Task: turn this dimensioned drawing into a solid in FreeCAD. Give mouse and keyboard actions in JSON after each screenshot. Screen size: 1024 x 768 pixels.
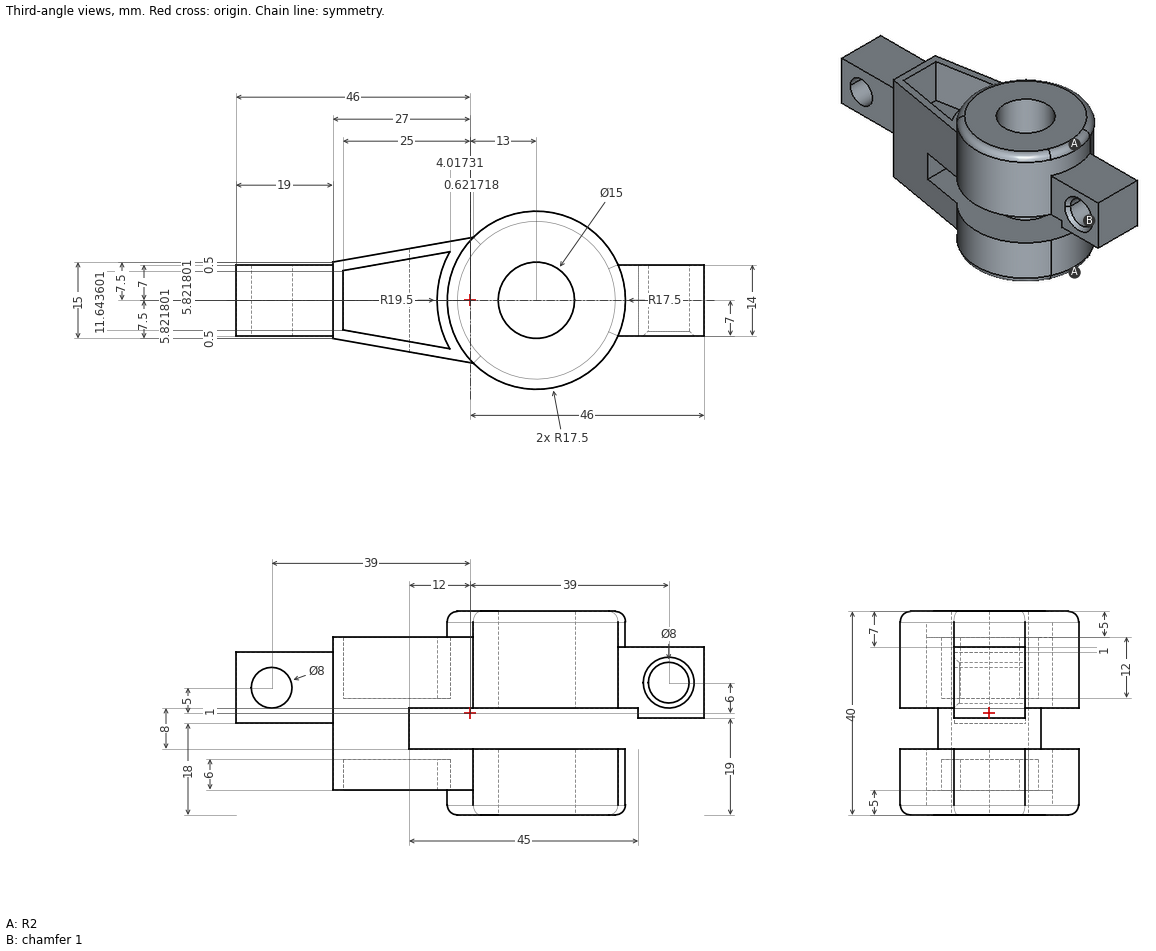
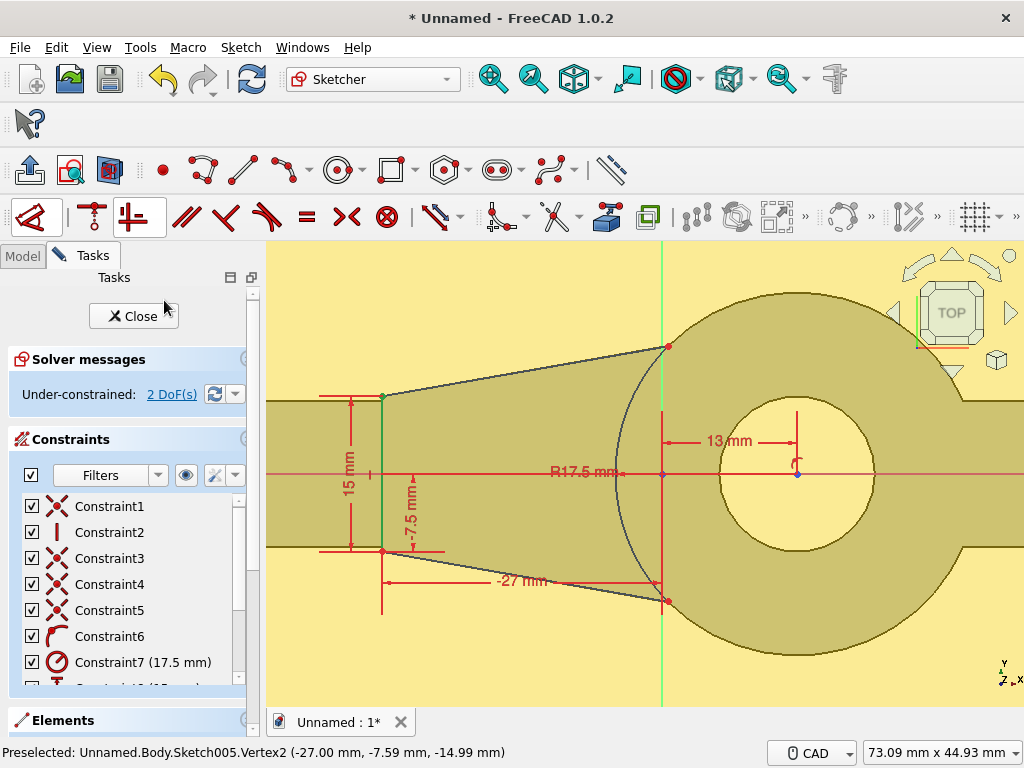
{"action": "scroll", "coordinate": [668, 602], "scroll_direction": "up", "scroll_amount": 10}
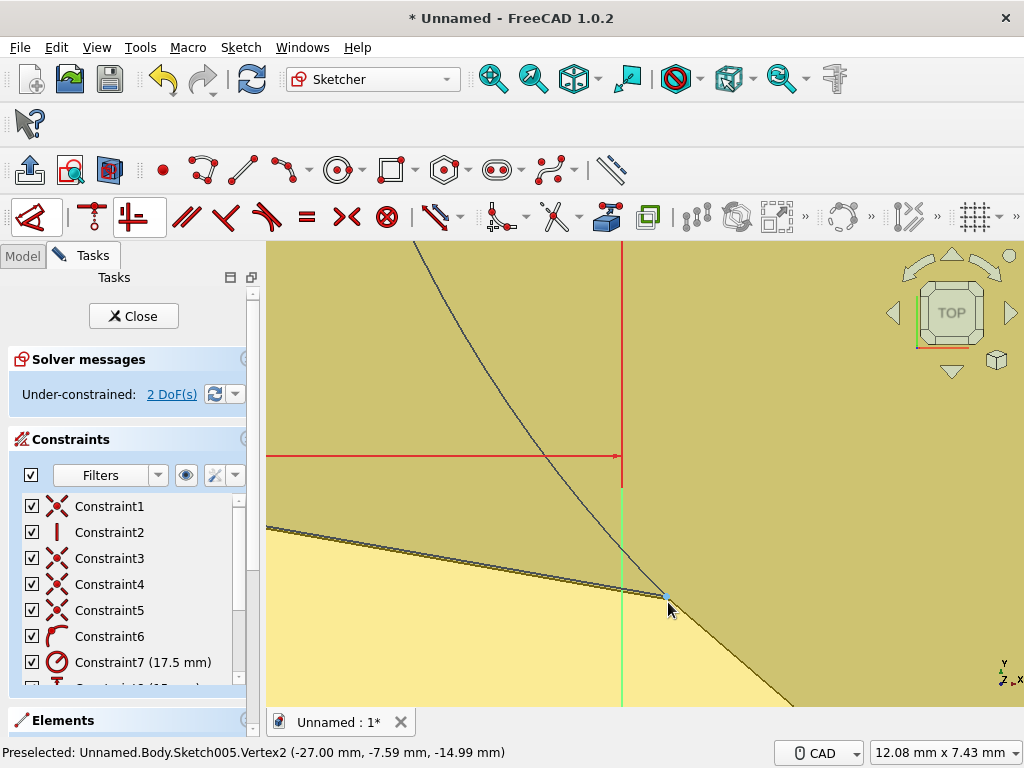
{"action": "left_click", "coordinate": [666, 596]}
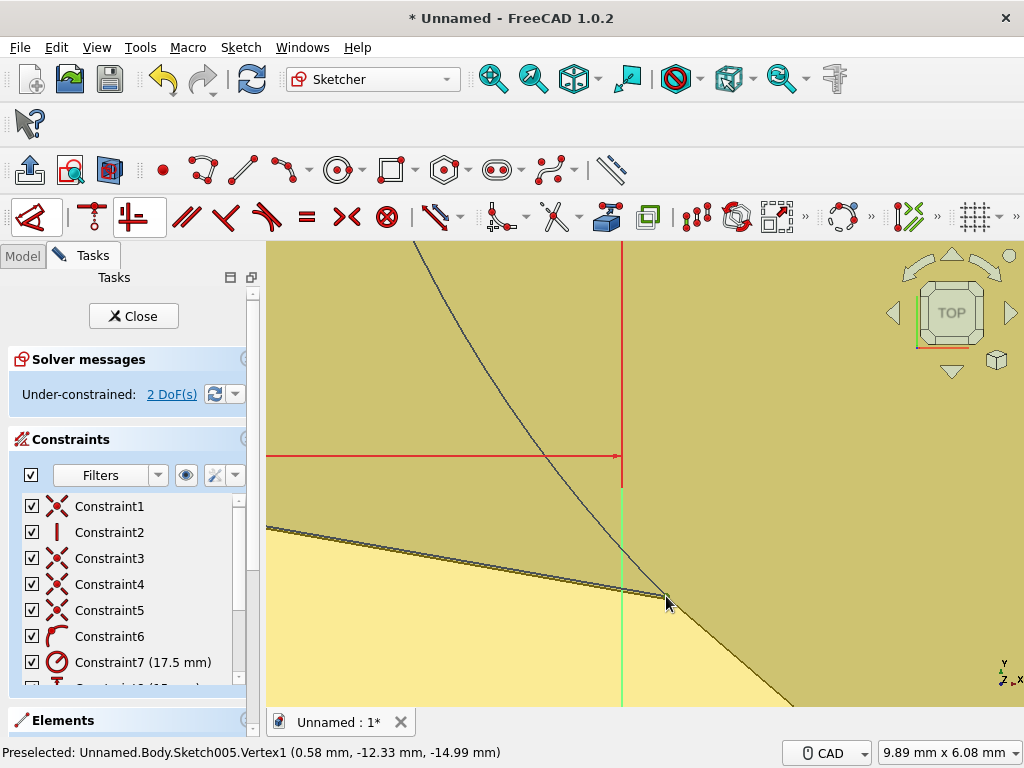
{"action": "key", "text": "l"}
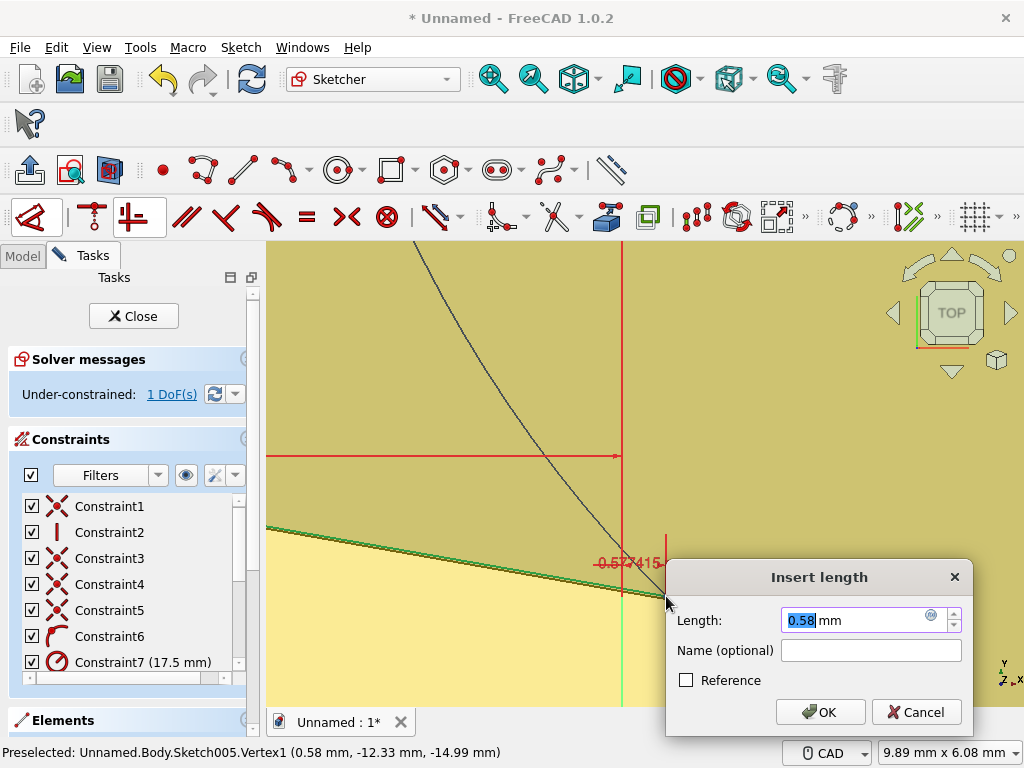
{"action": "type", "text": "0.621718"}
{"action": "key", "text": "Return"}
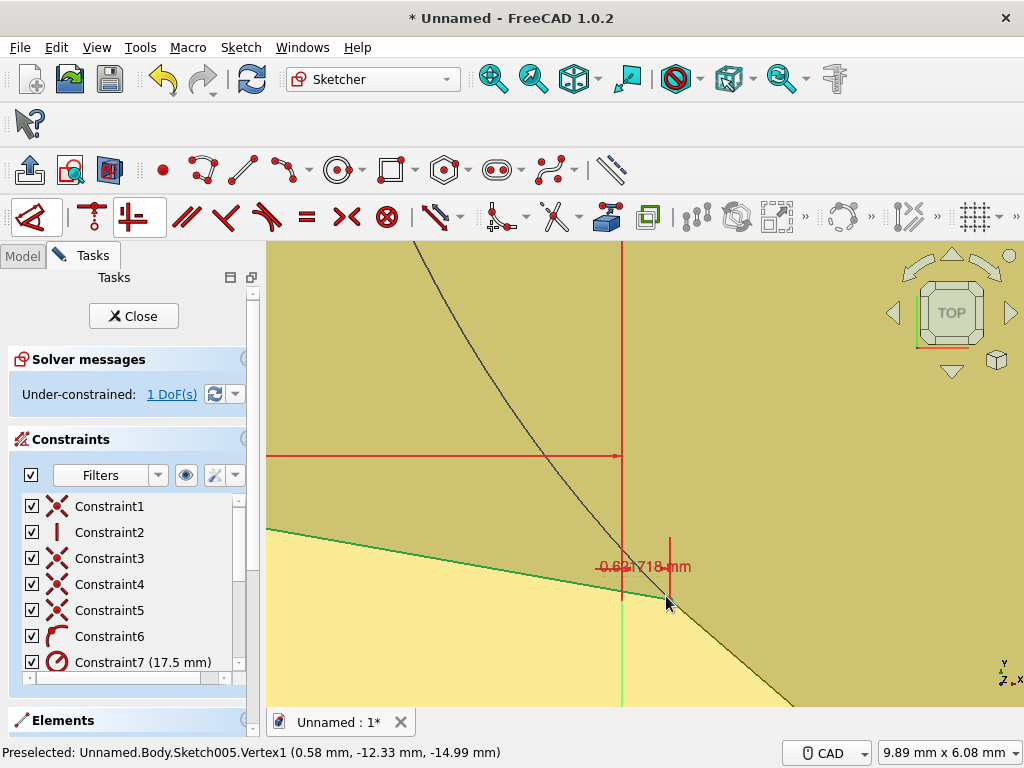
{"action": "scroll", "coordinate": [768, 637], "scroll_direction": "down", "scroll_amount": 9}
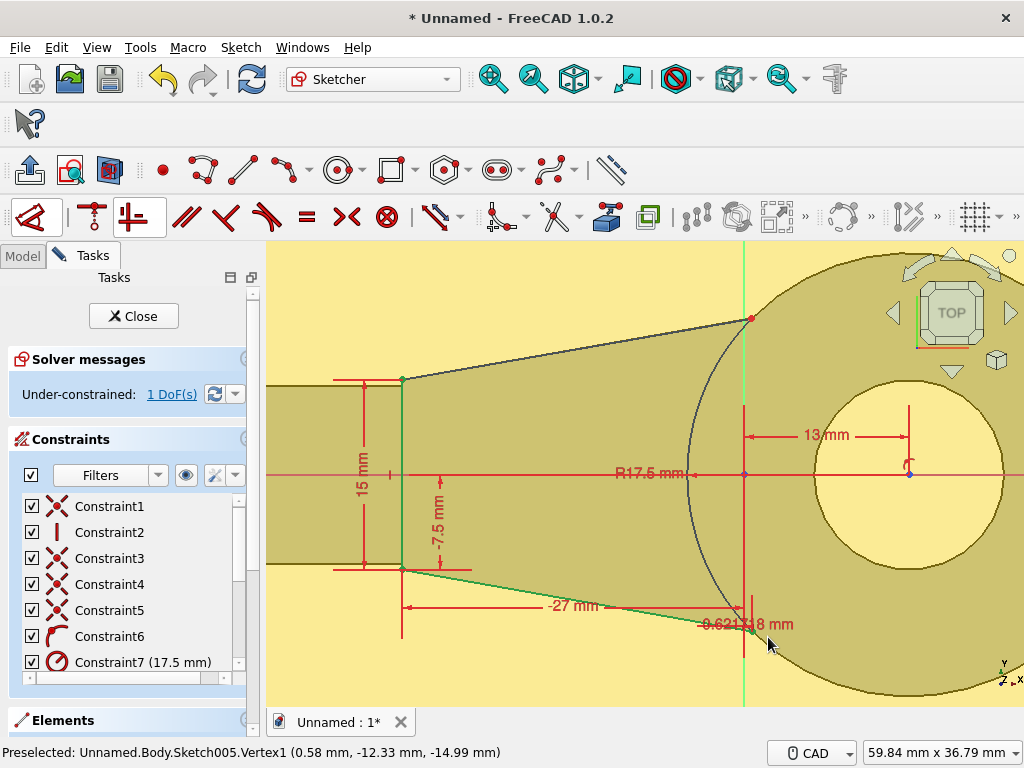
{"action": "scroll", "coordinate": [752, 319], "scroll_direction": "up", "scroll_amount": 9}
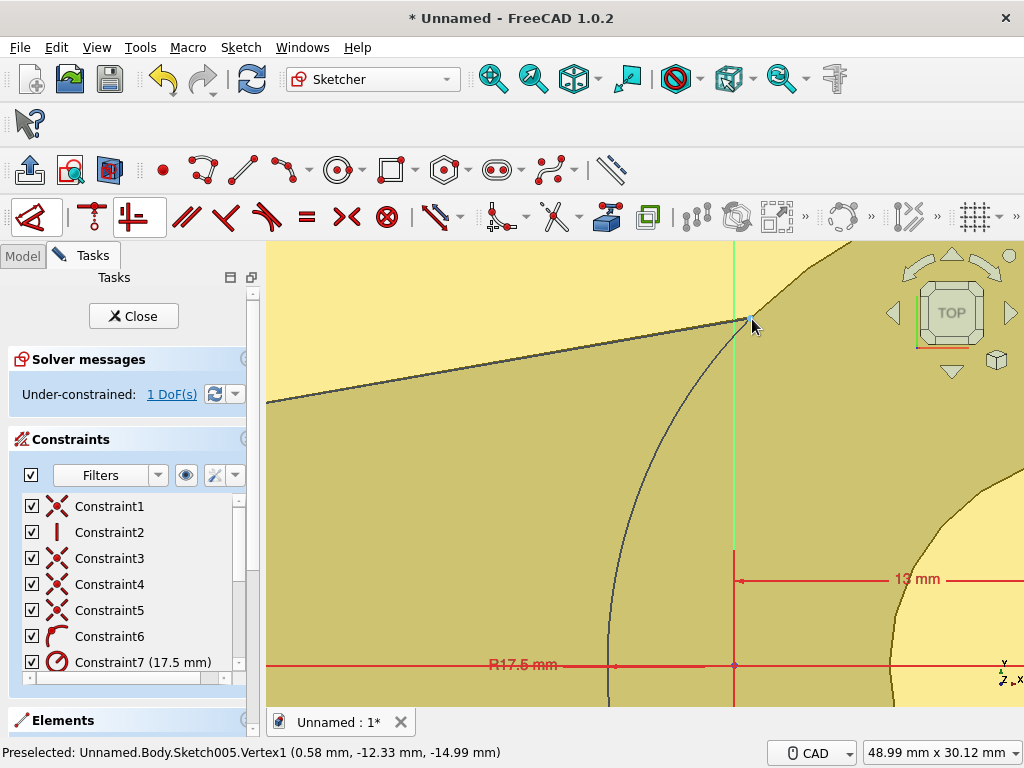
{"action": "left_click", "coordinate": [747, 317]}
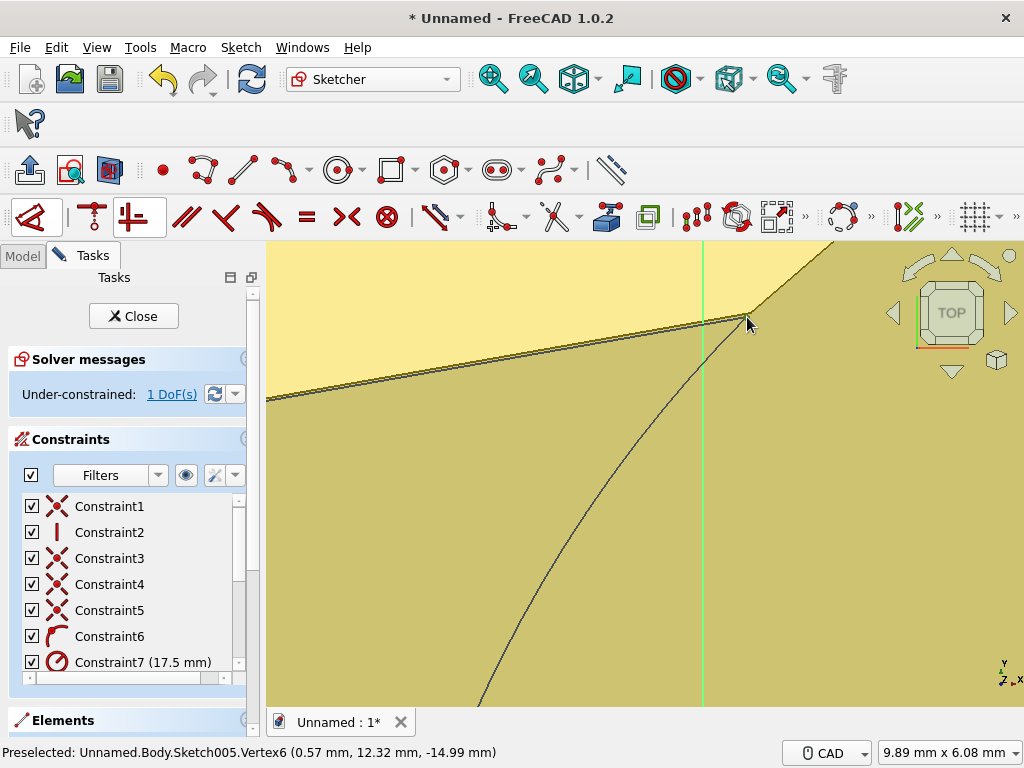
{"action": "key", "text": "l"}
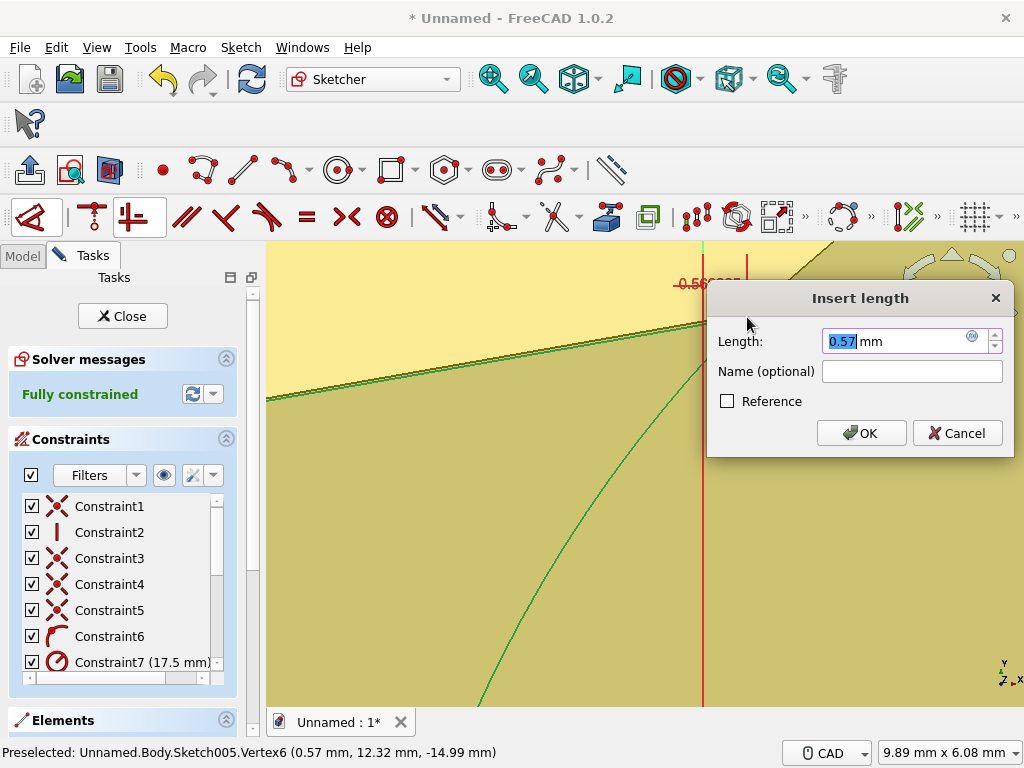
{"action": "type", "text": "0.621718"}
{"action": "key", "text": "Return"}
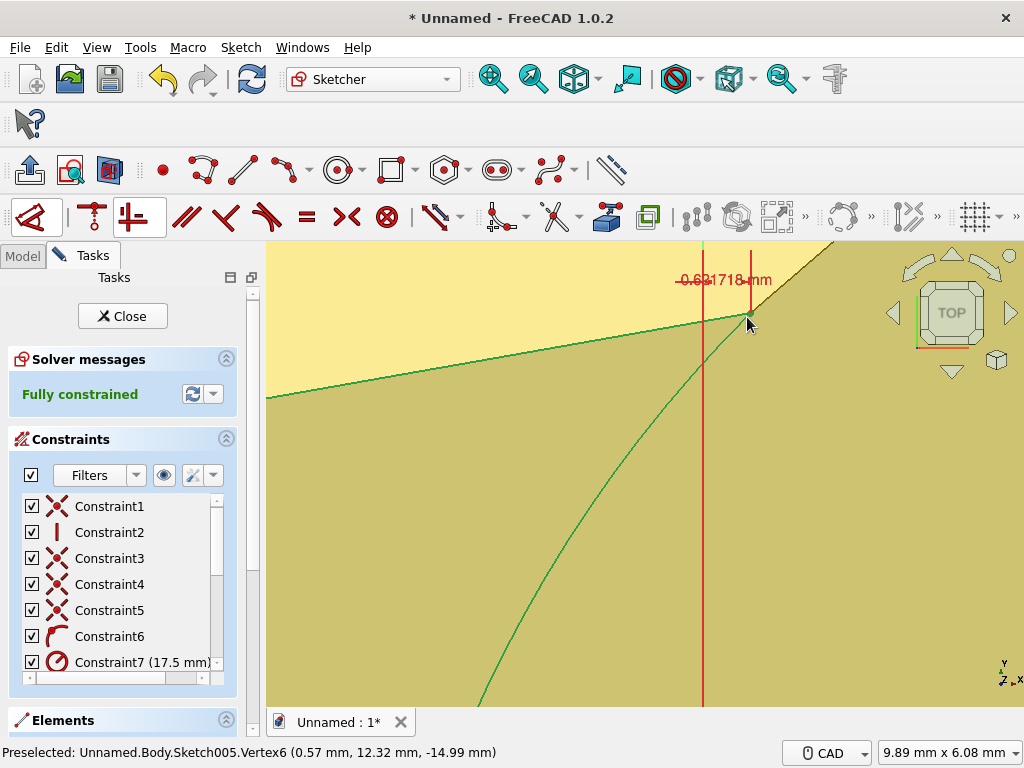
{"action": "left_click", "coordinate": [123, 316]}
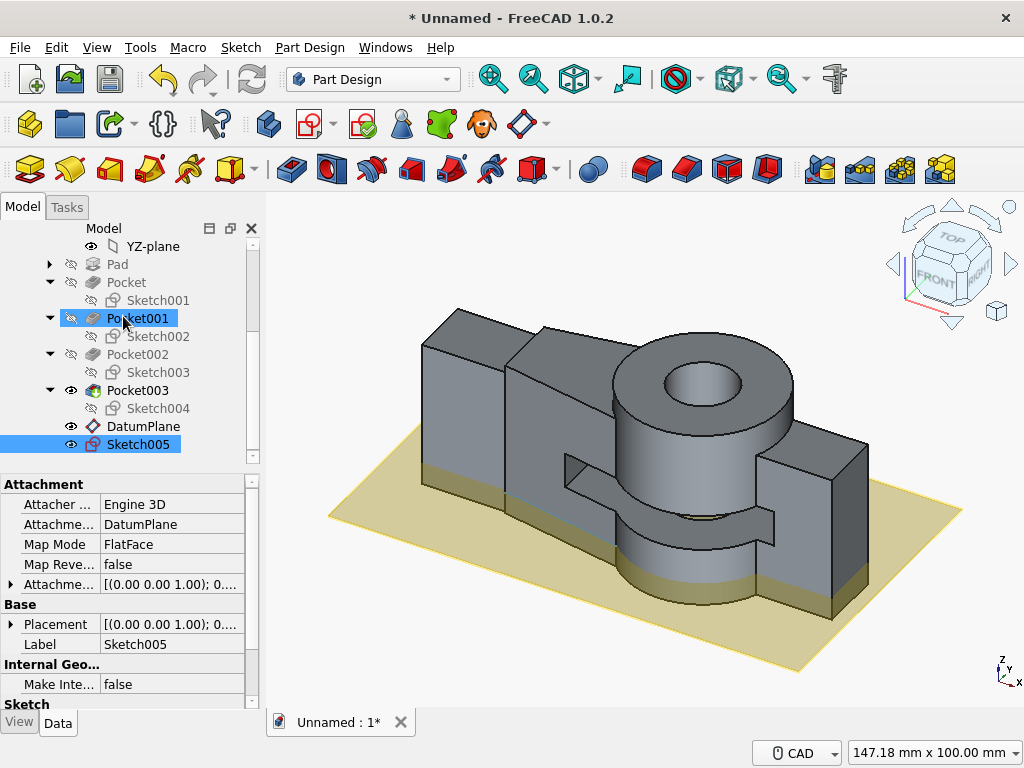
{"action": "left_click", "coordinate": [292, 170]}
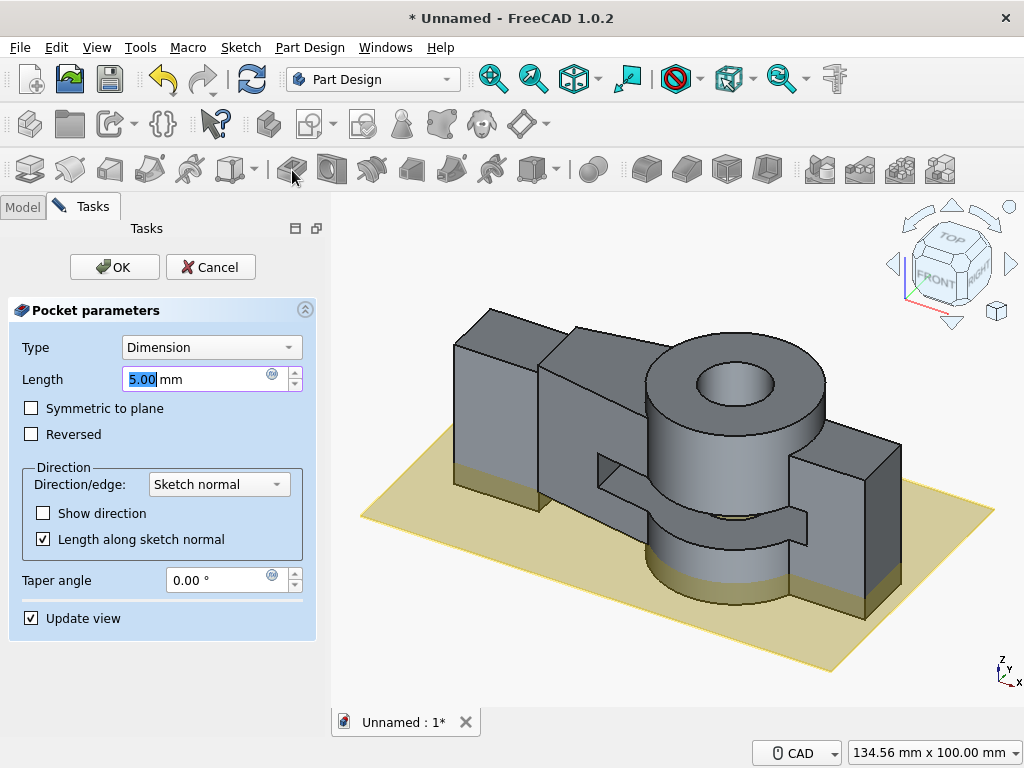
{"action": "type", "text": "5"}
{"action": "key", "text": "Tab"}